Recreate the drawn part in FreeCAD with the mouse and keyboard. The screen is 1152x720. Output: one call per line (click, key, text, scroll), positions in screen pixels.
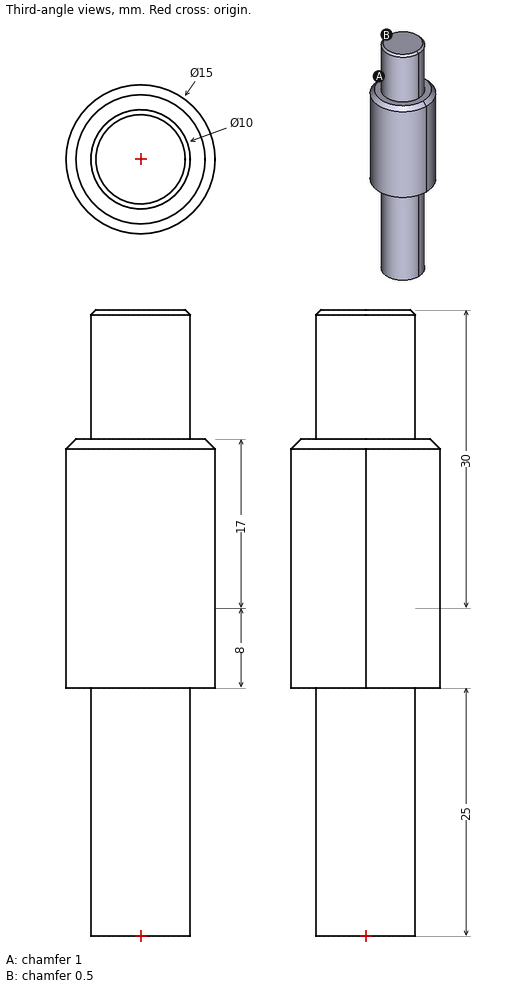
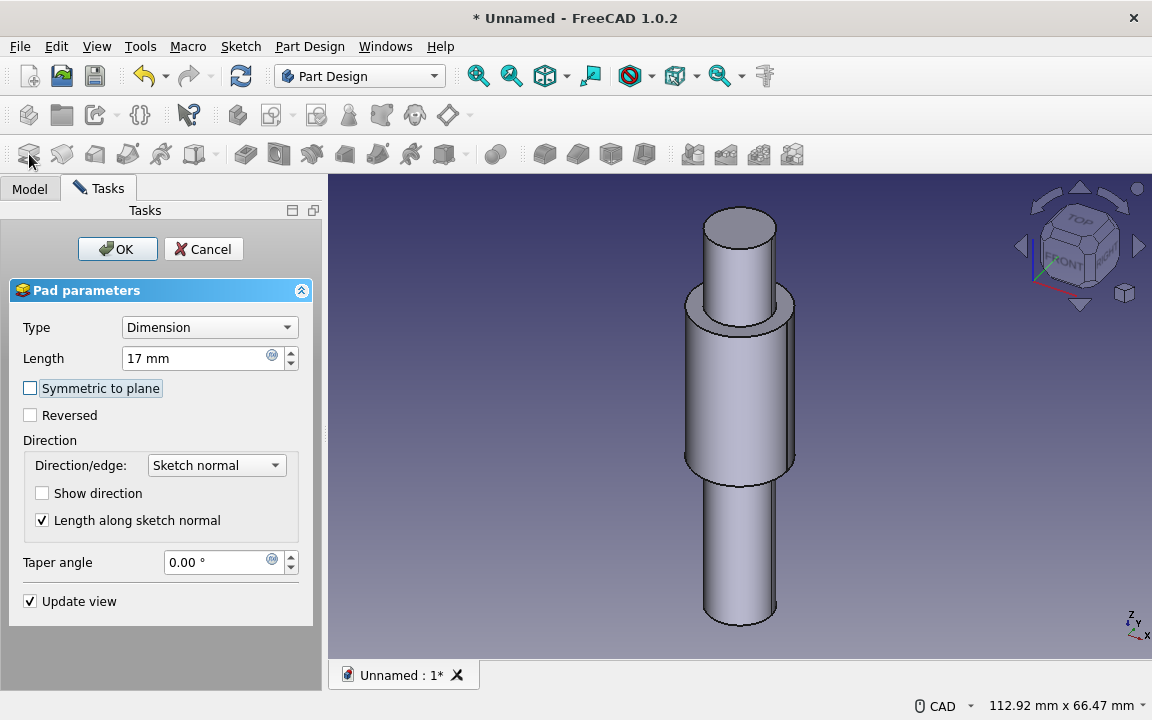
click(118, 249)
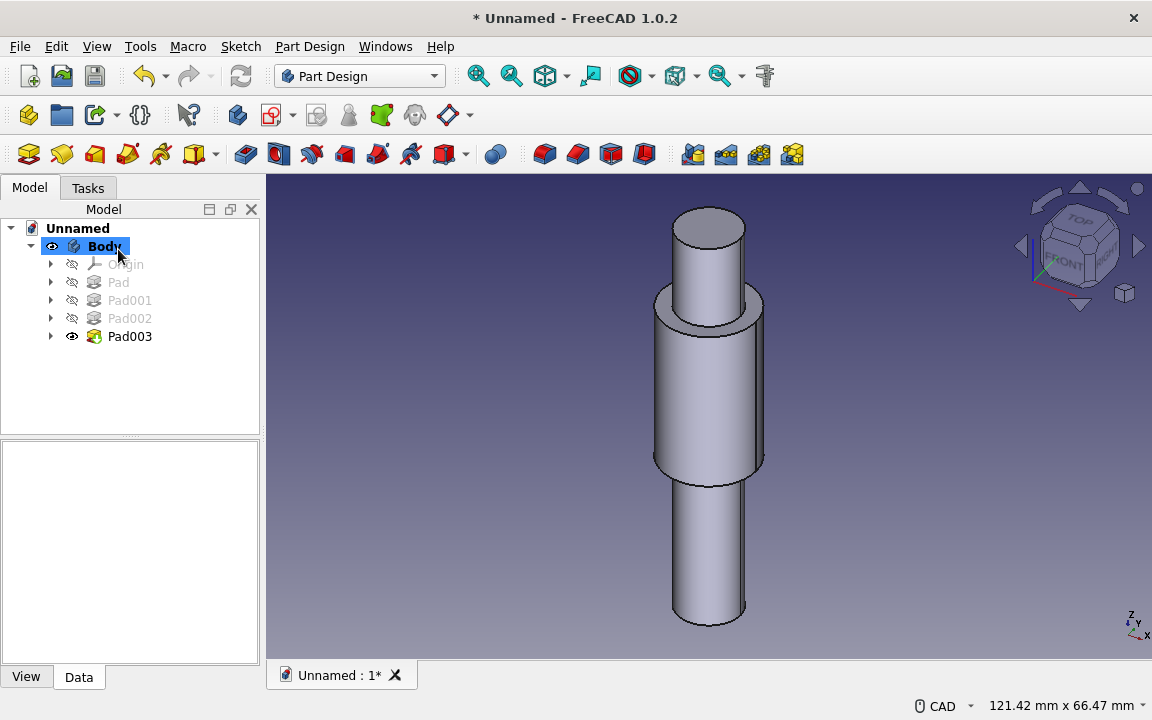
click(654, 308)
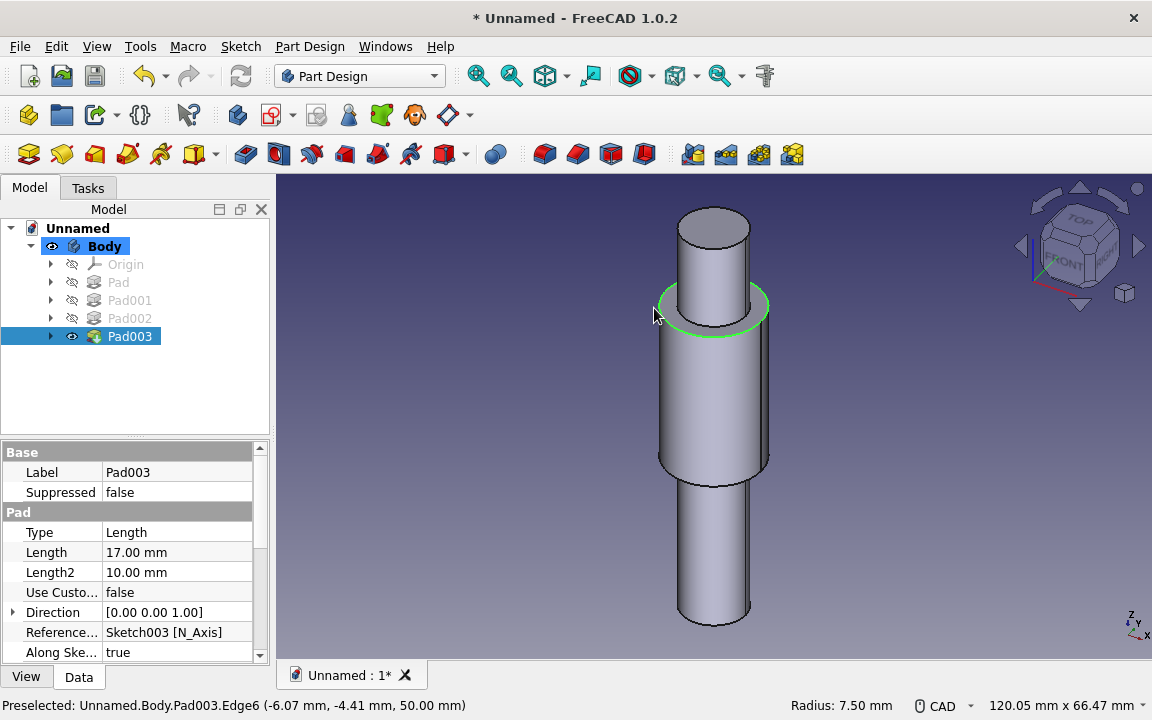
click(578, 154)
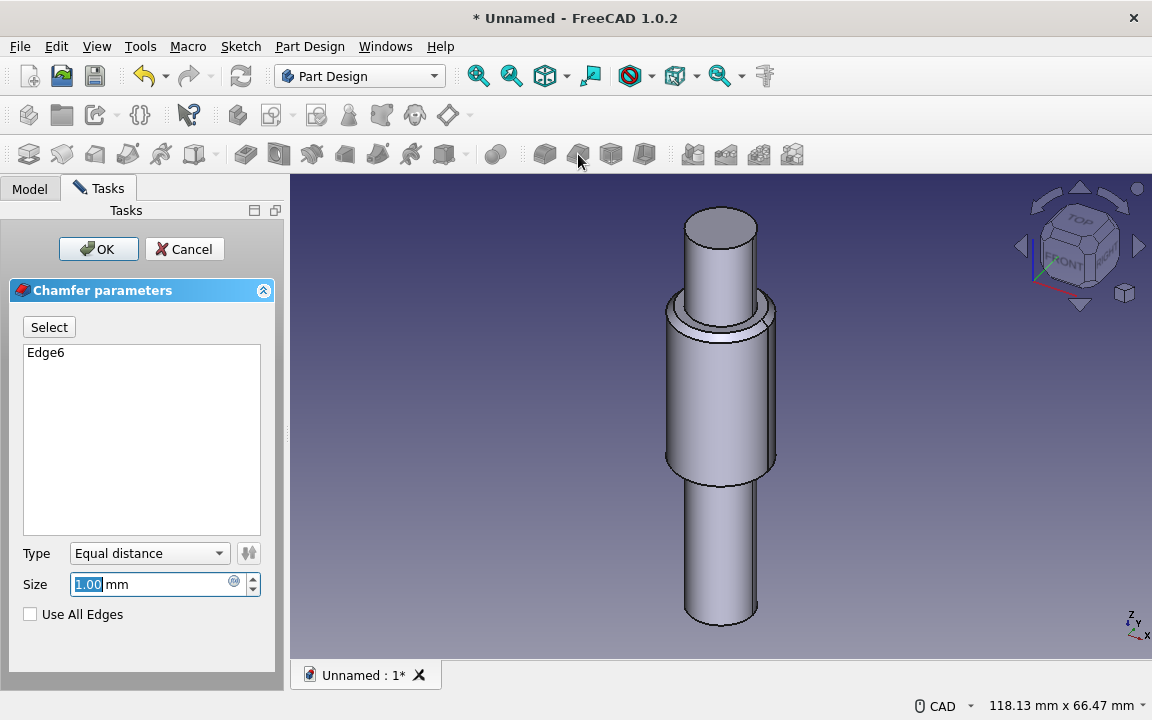
text(1)
key(Tab)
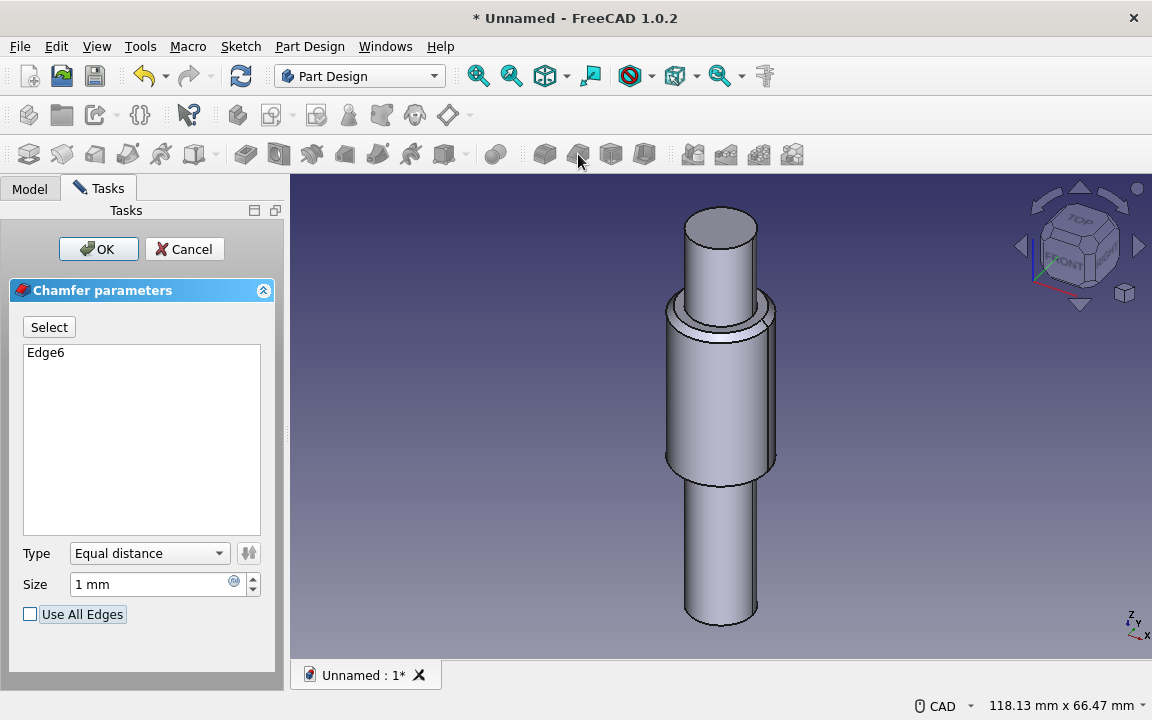
click(99, 249)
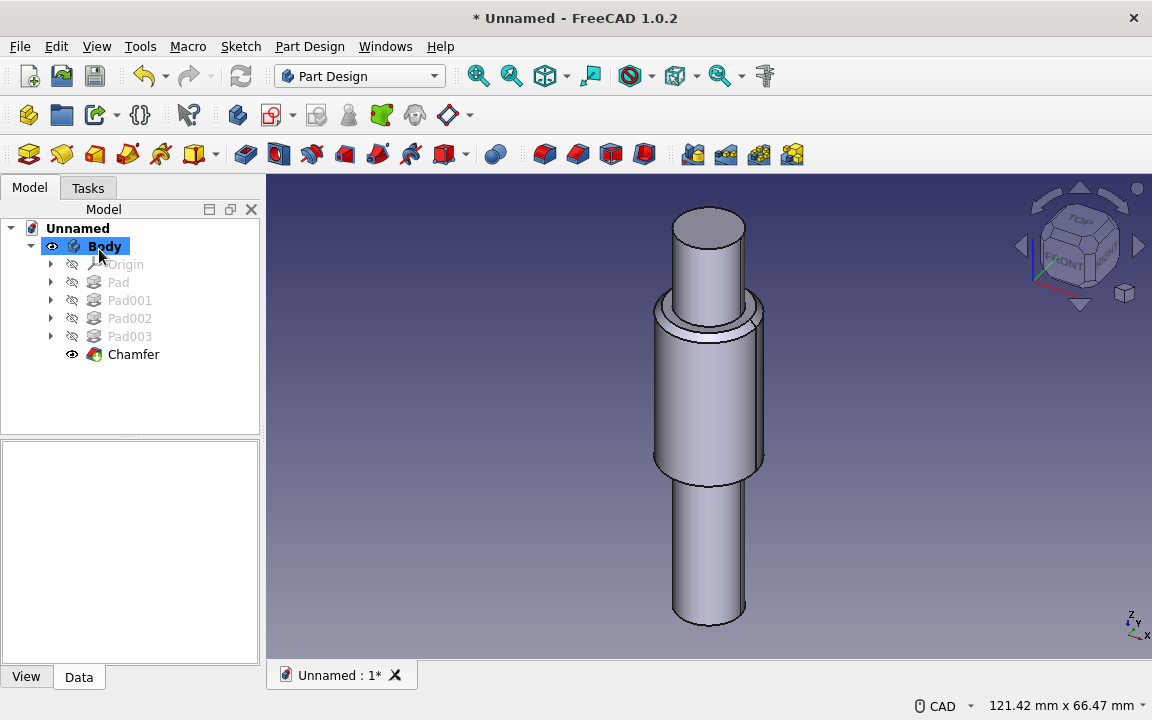
click(677, 217)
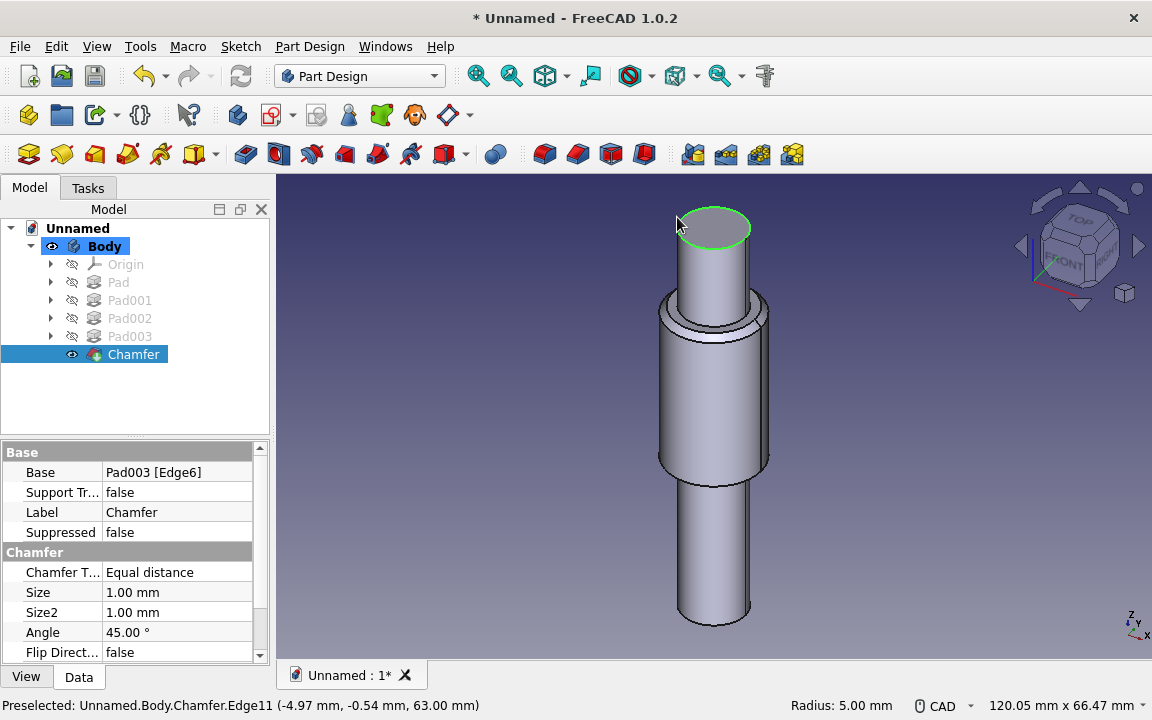
click(578, 154)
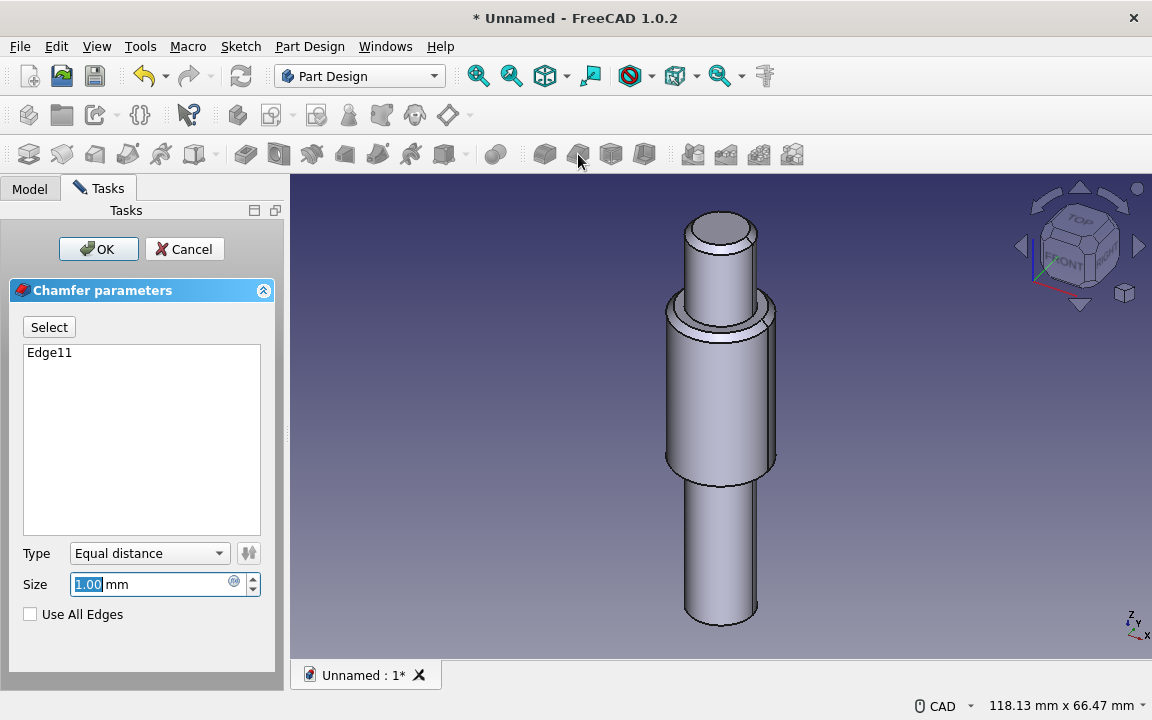
text(0.5)
key(Tab)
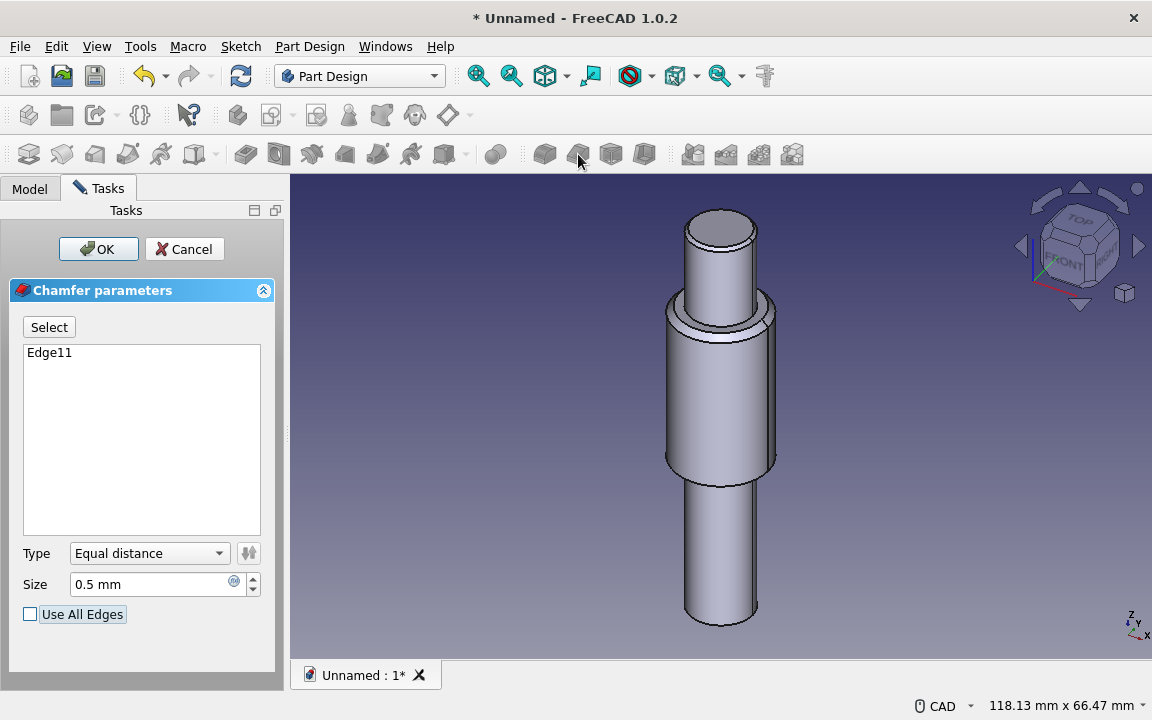
click(99, 249)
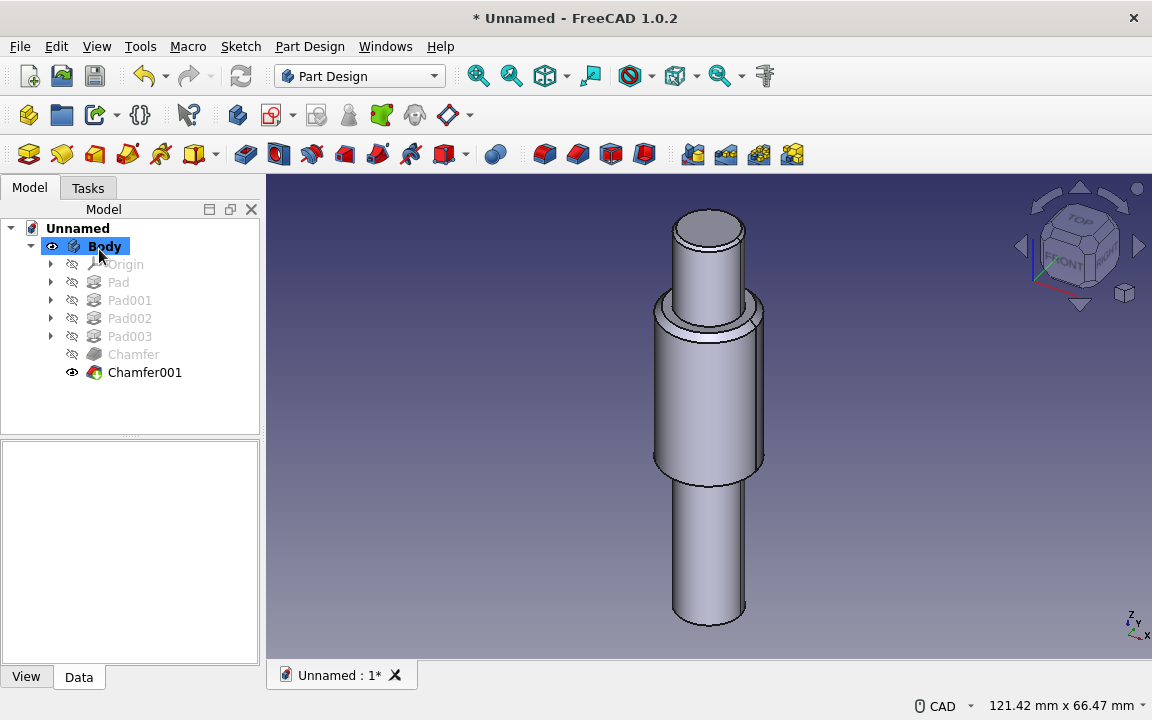
key(0)